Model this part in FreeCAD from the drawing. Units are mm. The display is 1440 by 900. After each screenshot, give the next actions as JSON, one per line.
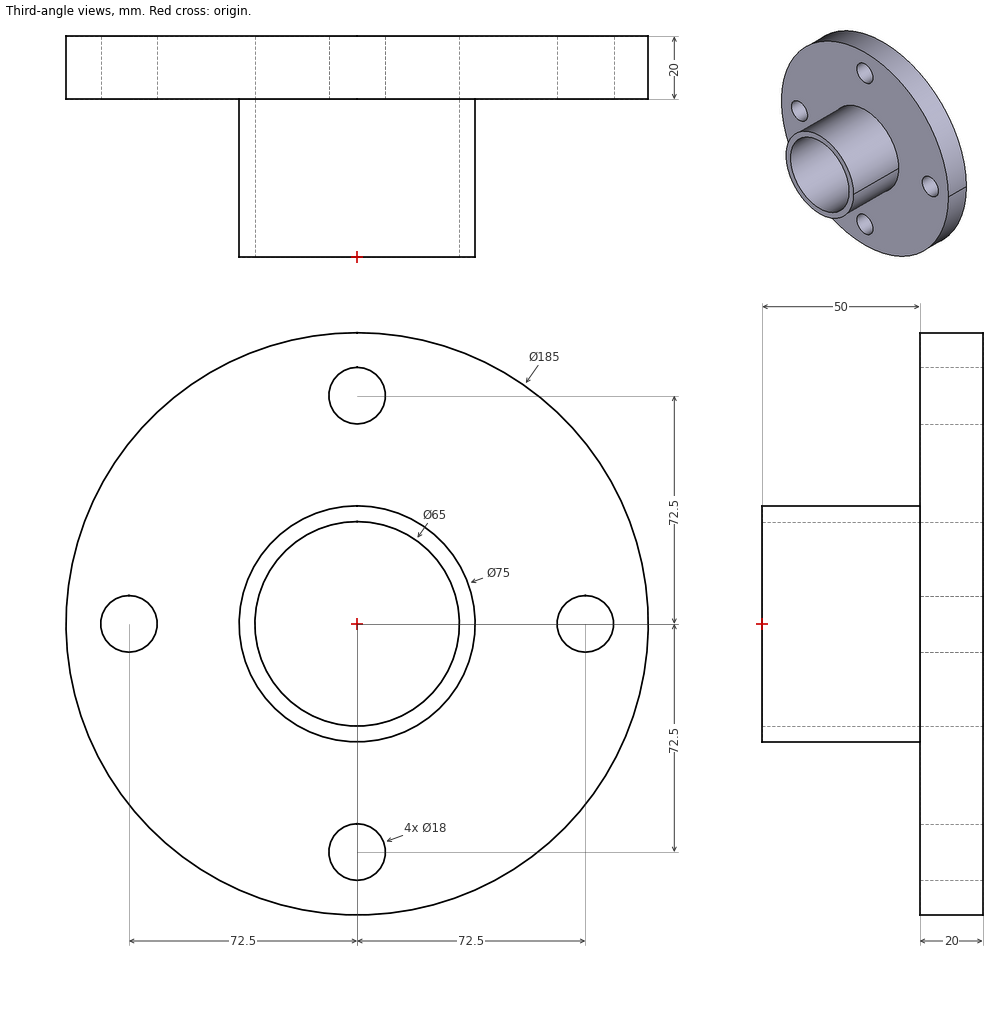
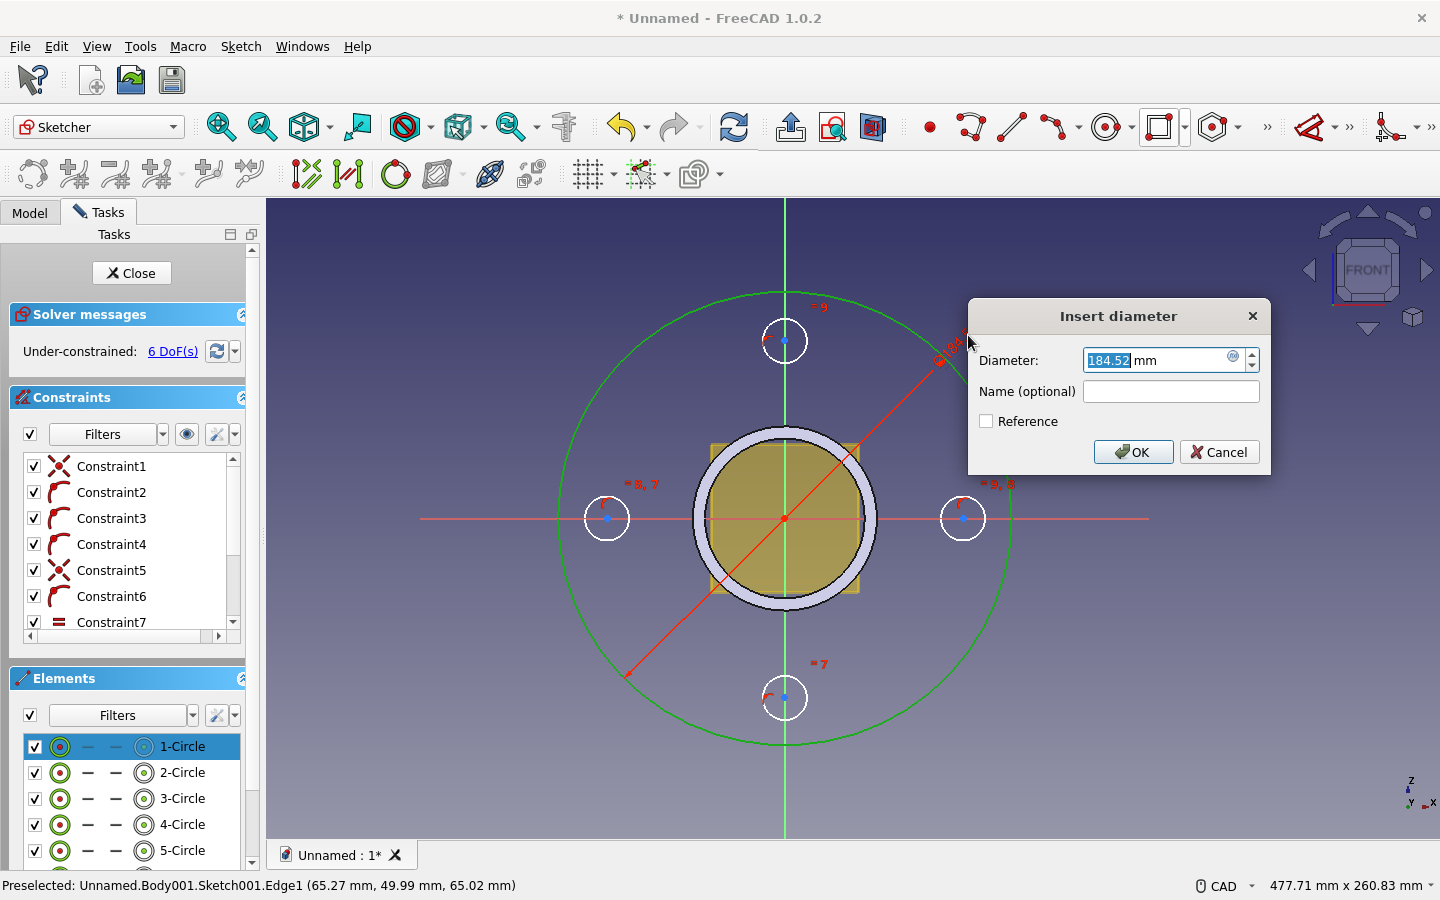
{"action": "type", "text": "185"}
{"action": "key", "text": "Return"}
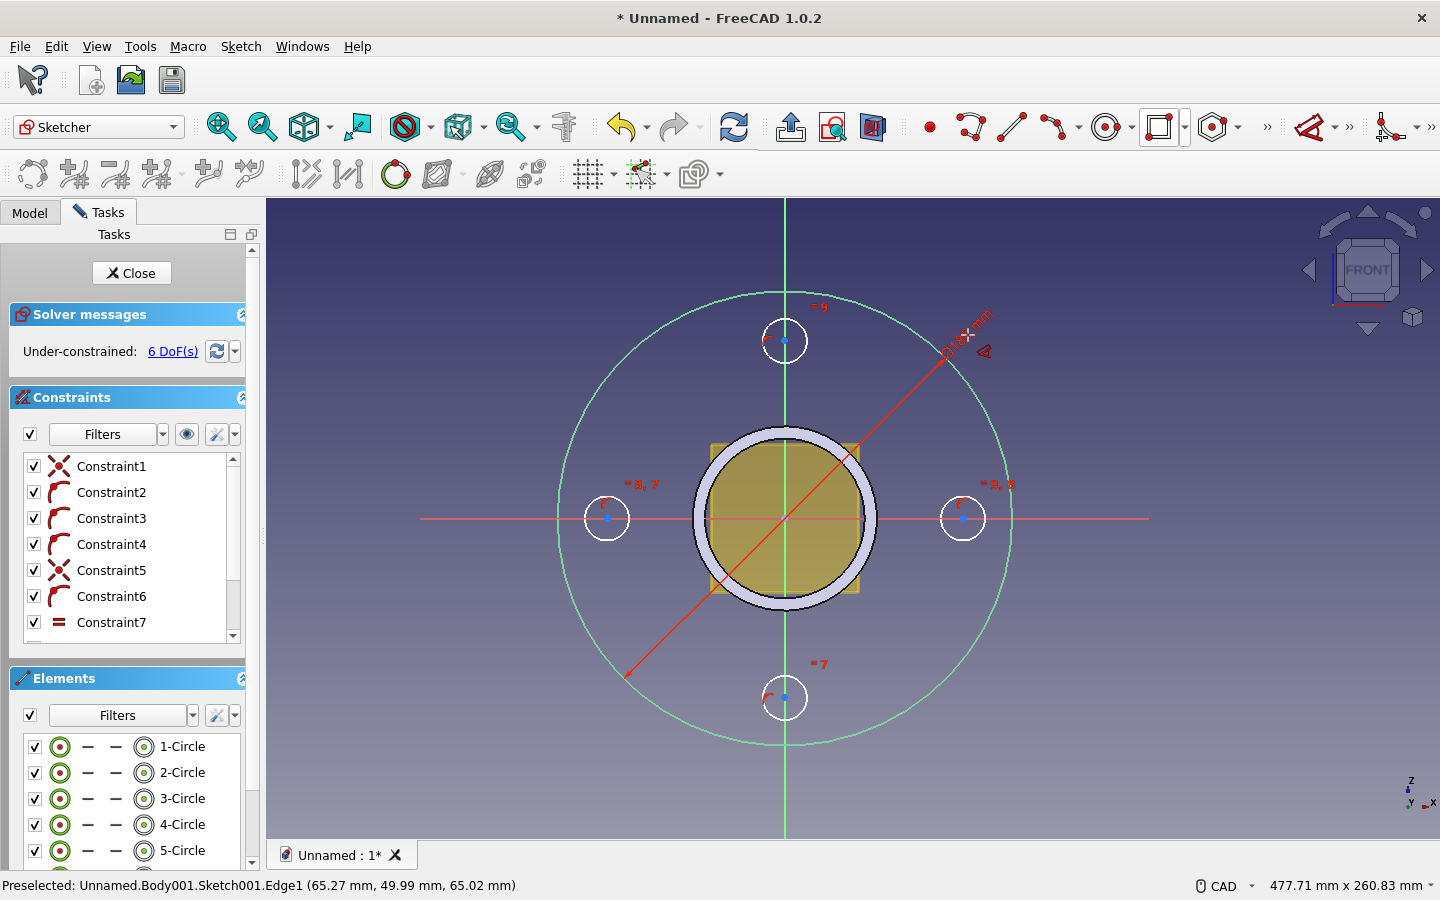
{"action": "left_click", "coordinate": [800, 682]}
{"action": "left_click", "coordinate": [822, 659]}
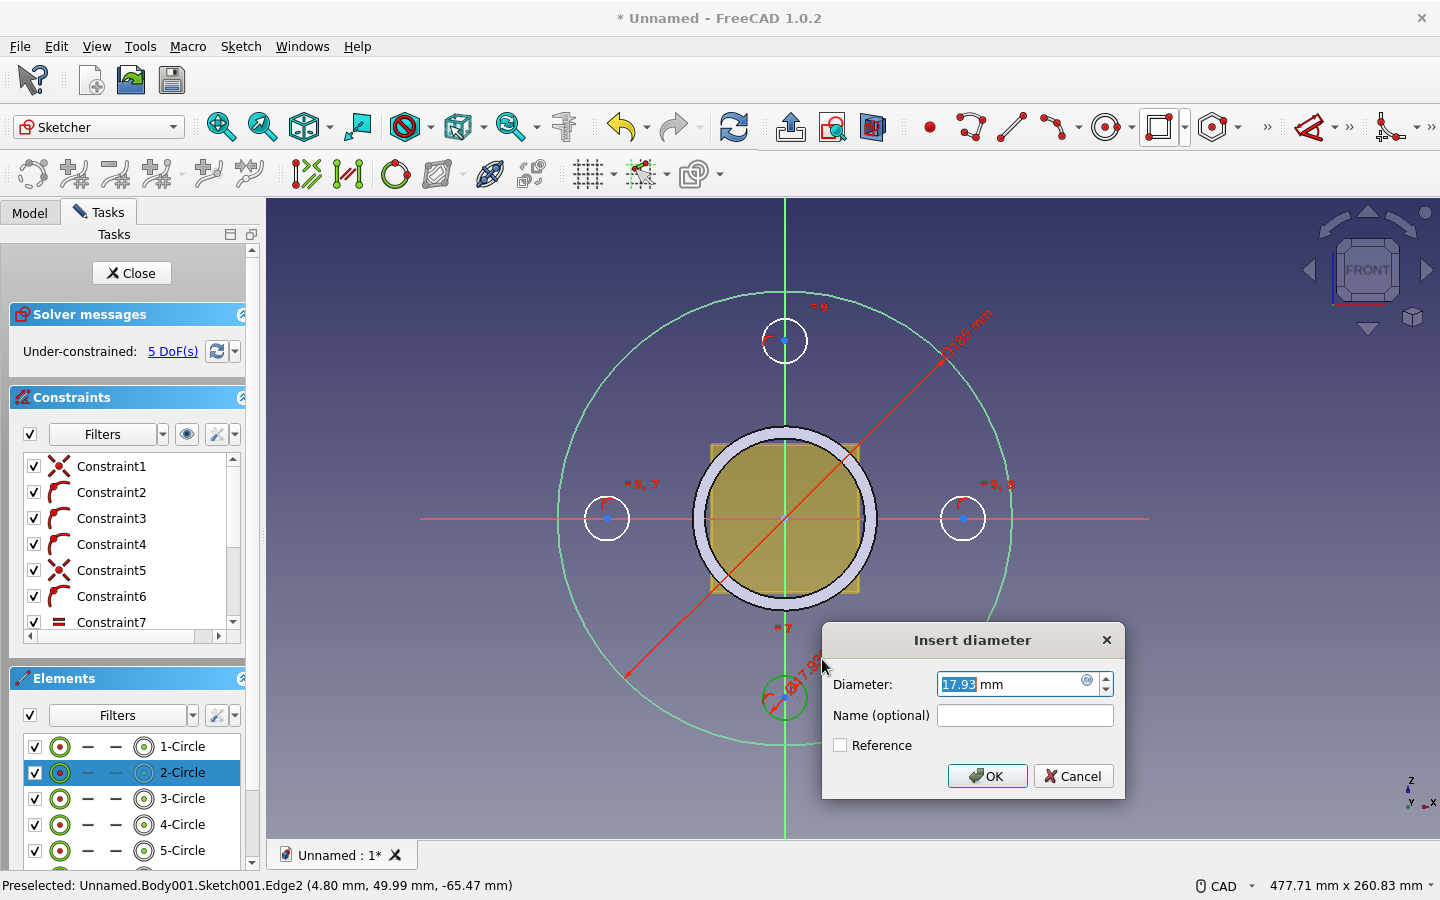
{"action": "type", "text": "18"}
{"action": "key", "text": "Return"}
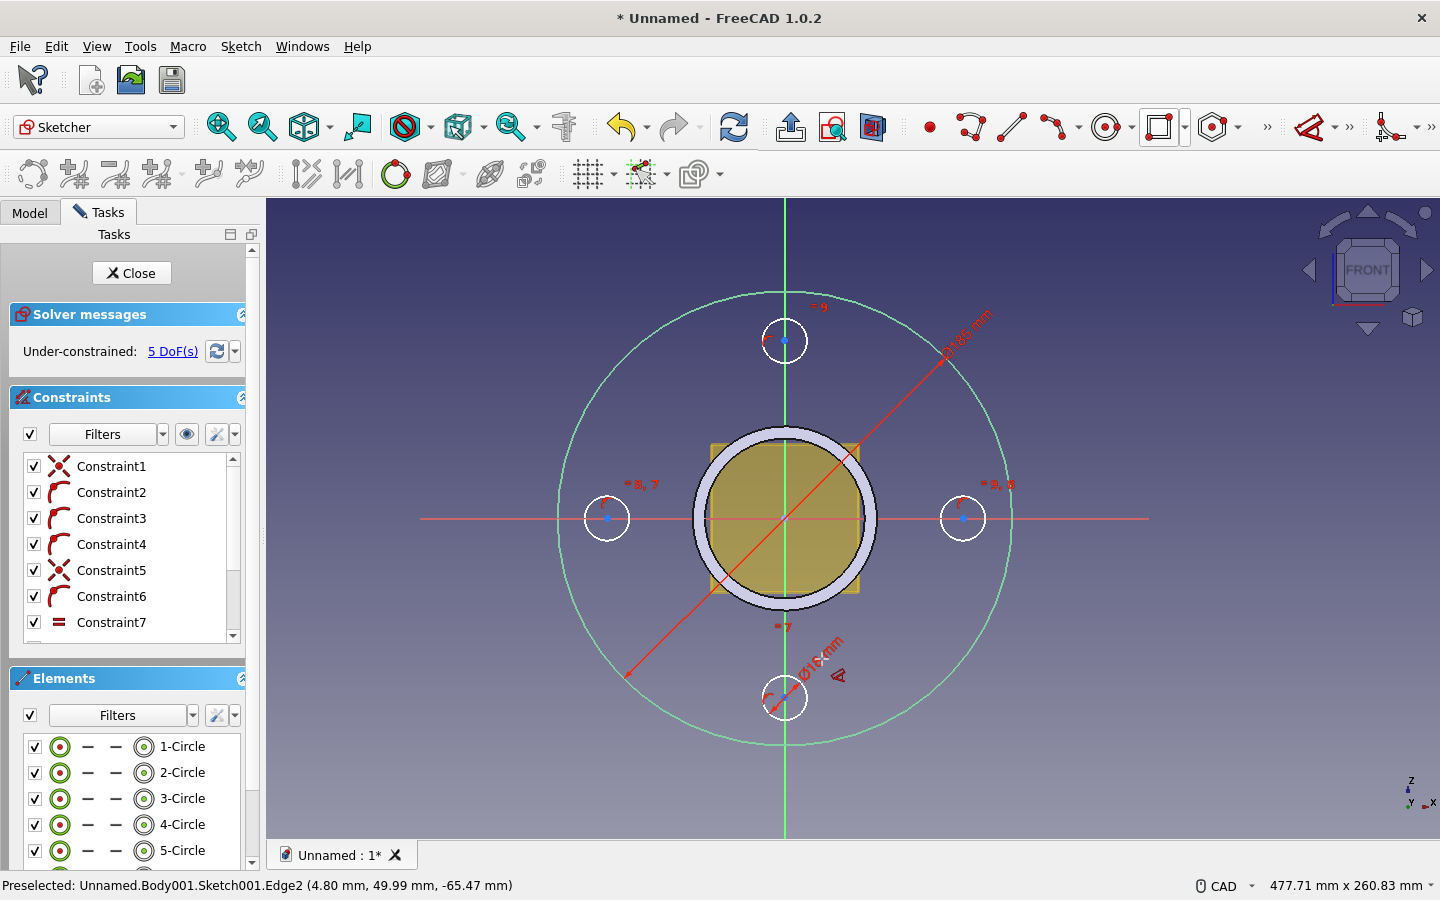
{"action": "left_click", "coordinate": [849, 453]}
{"action": "left_click", "coordinate": [871, 430]}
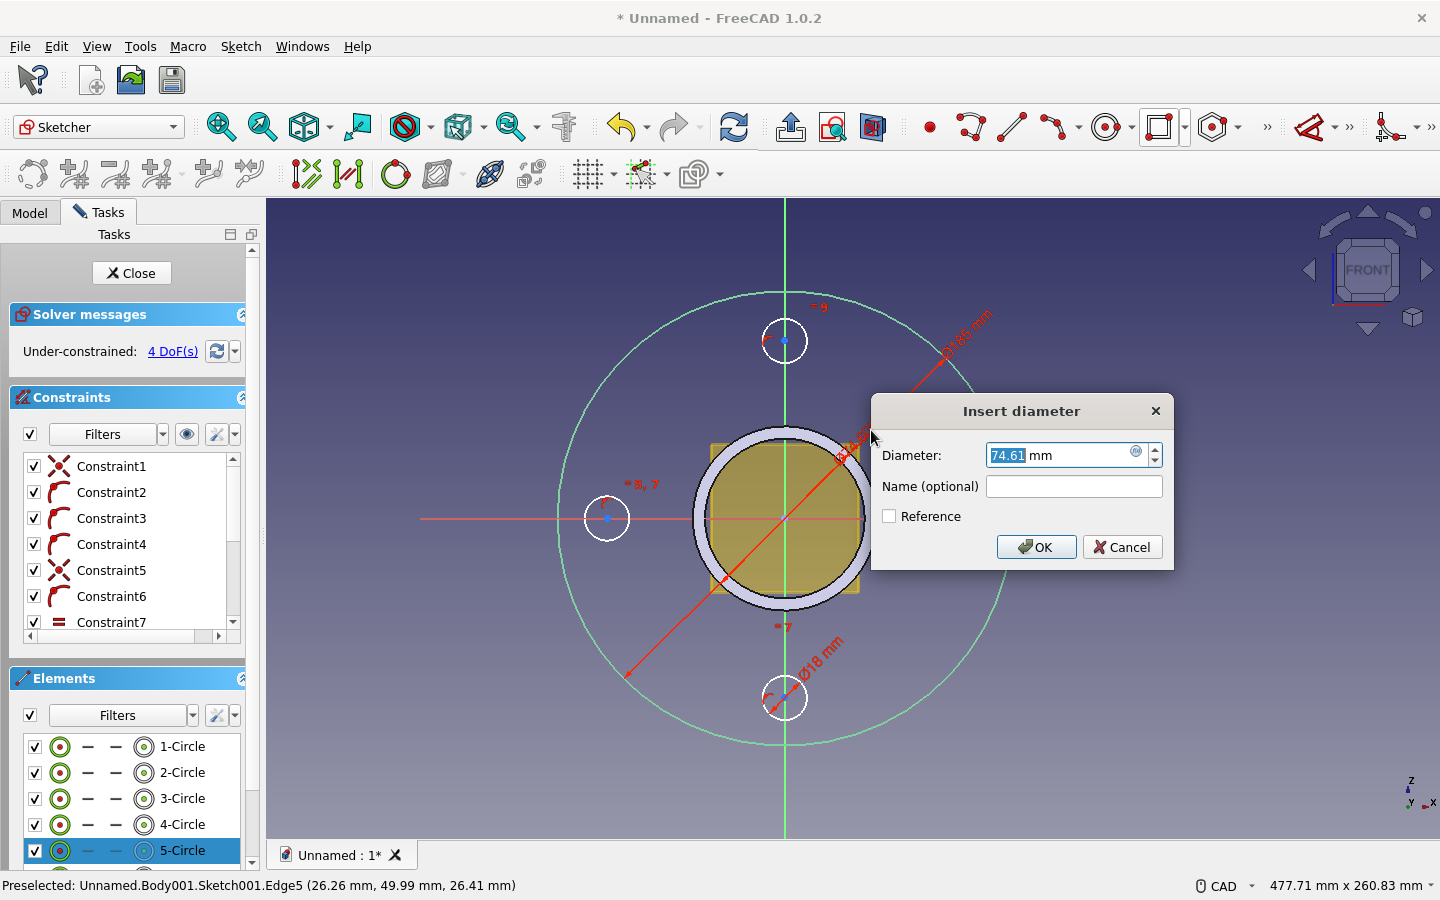
{"action": "type", "text": "75"}
{"action": "key", "text": "Return"}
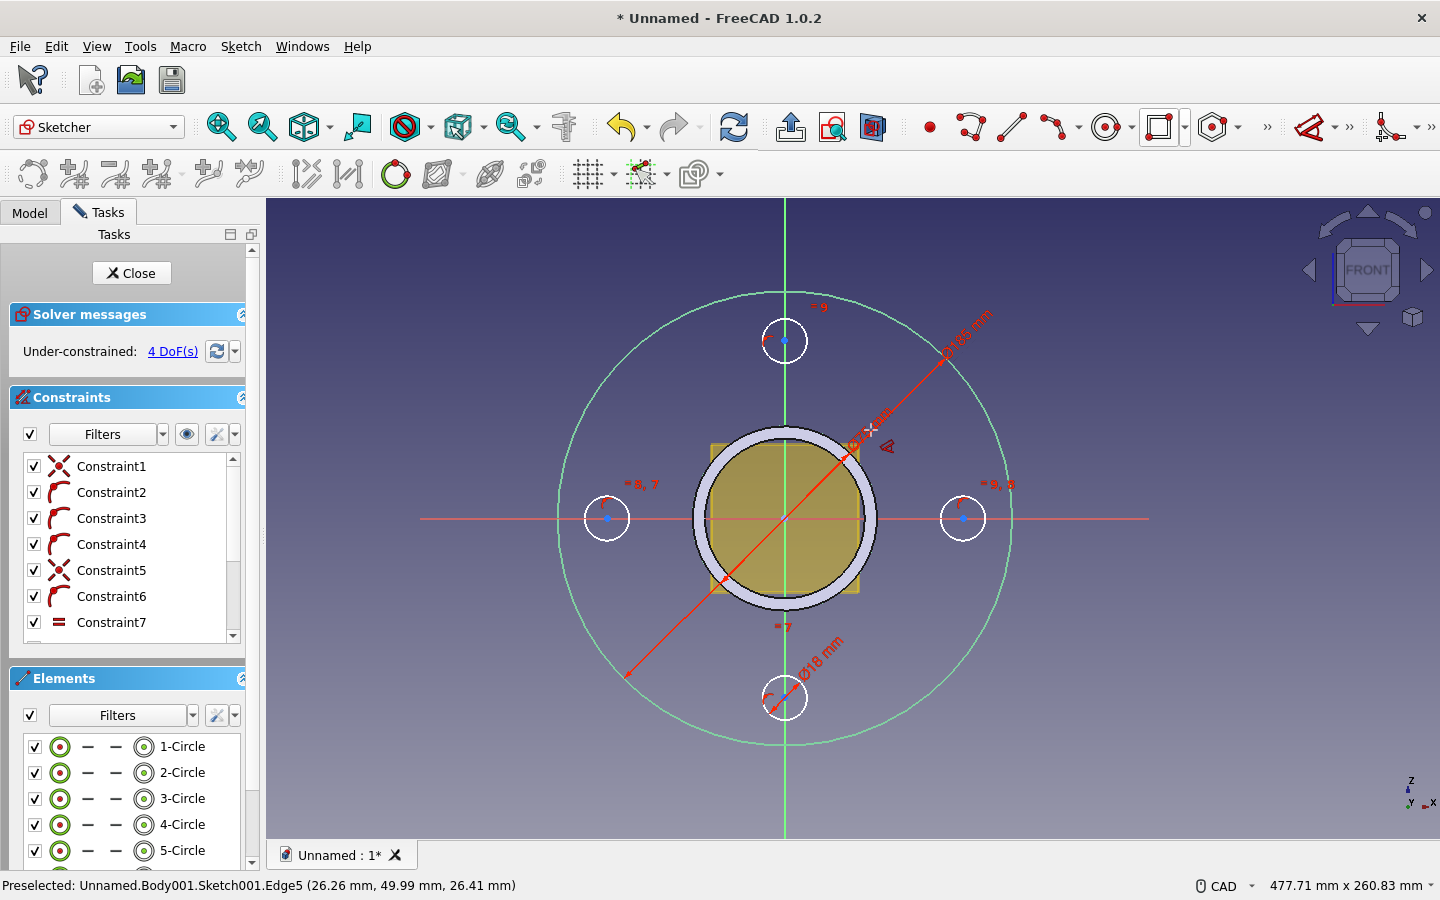
{"action": "left_click", "coordinate": [785, 698]}
{"action": "left_click", "coordinate": [819, 567]}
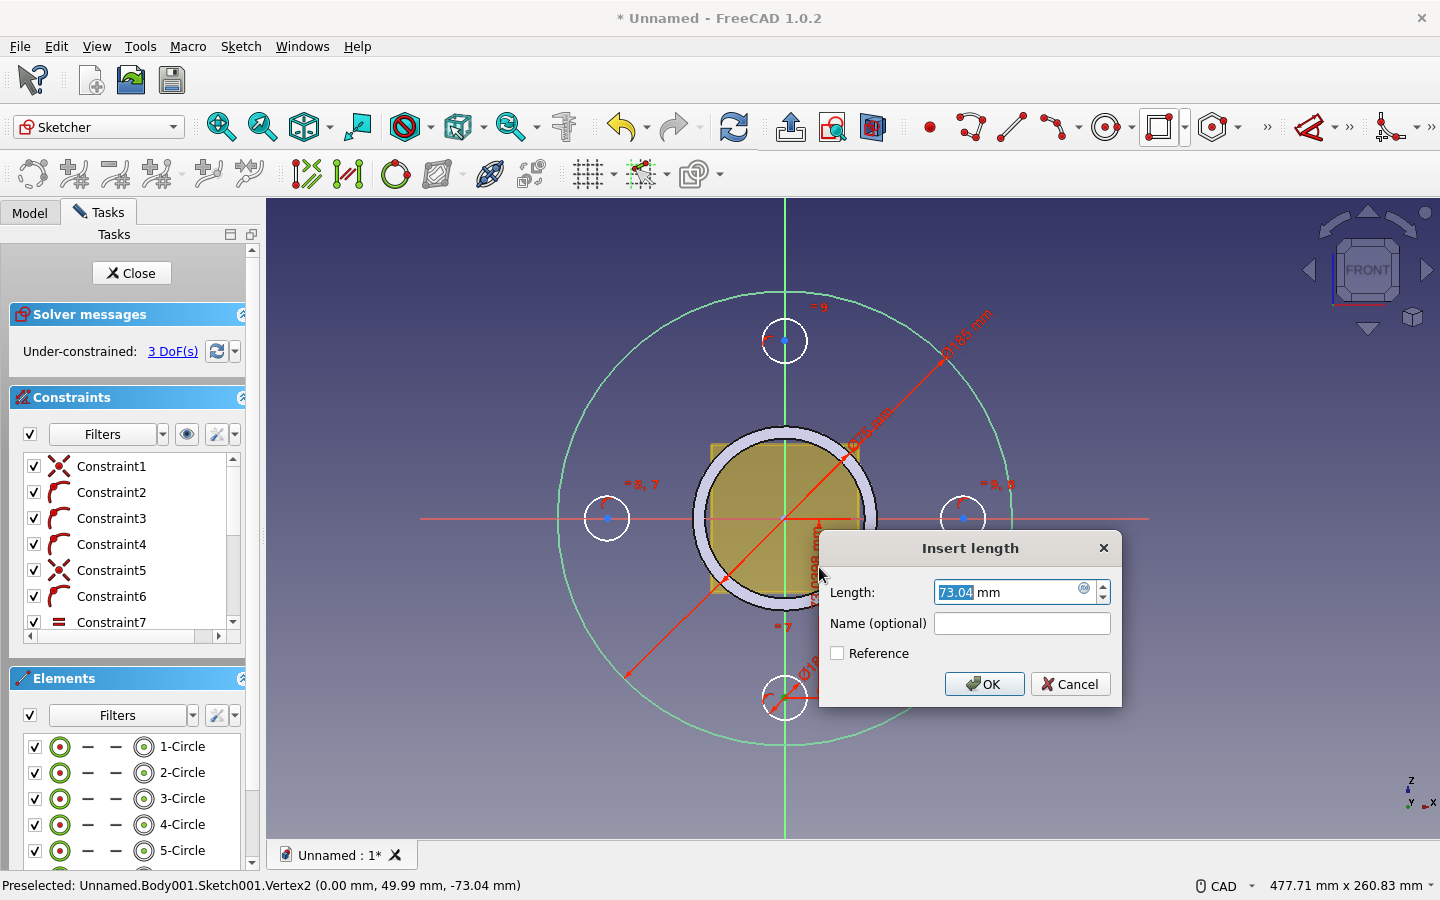
{"action": "type", "text": "72.5"}
{"action": "key", "text": "Return"}